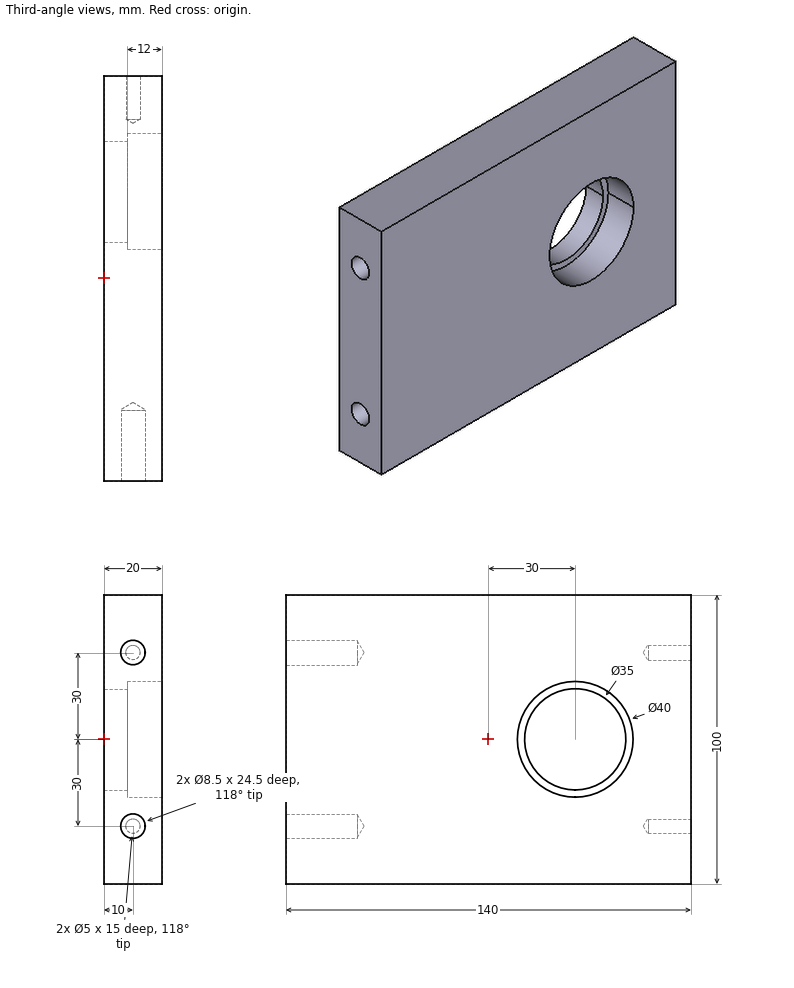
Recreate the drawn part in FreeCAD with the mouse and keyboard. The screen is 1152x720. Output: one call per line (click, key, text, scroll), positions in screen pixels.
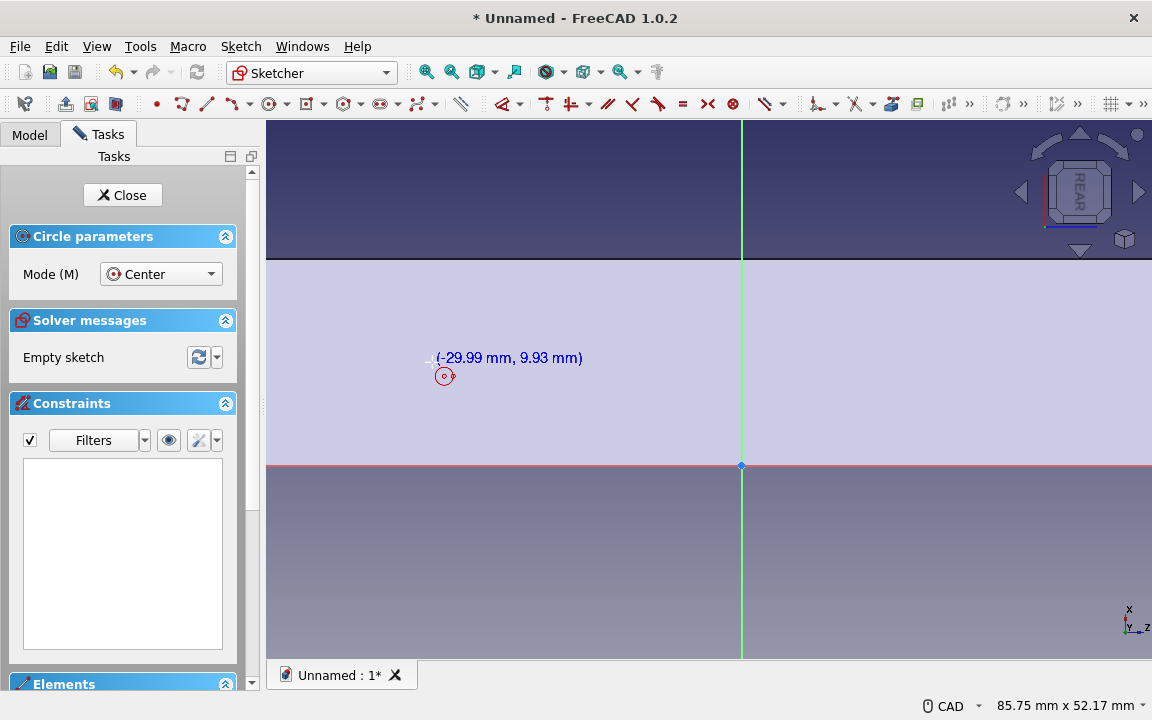
click(432, 363)
move(450, 344)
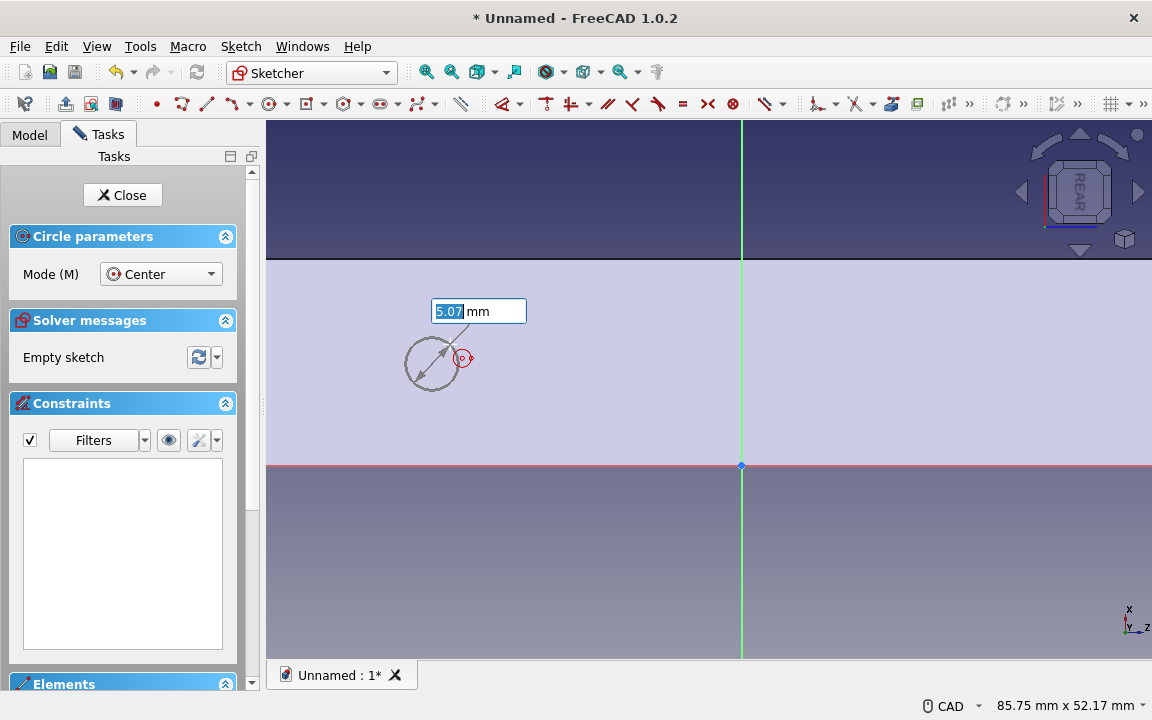
text(5)
key(Return)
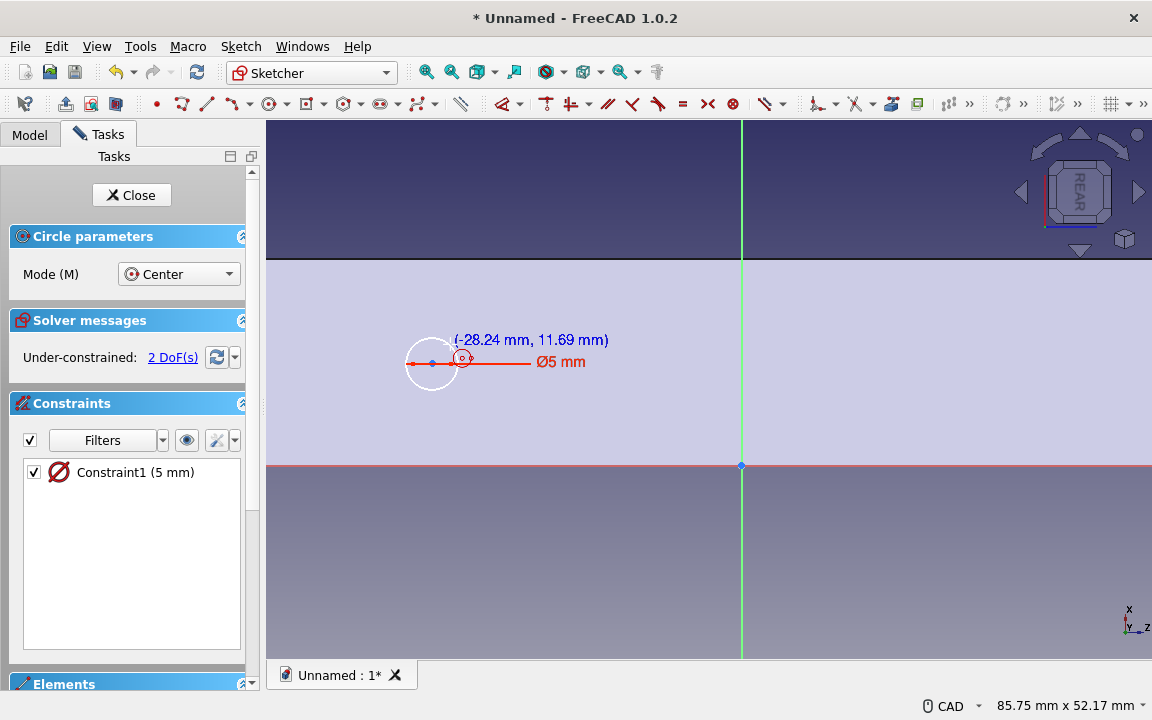
scroll(435, 366, down, 2)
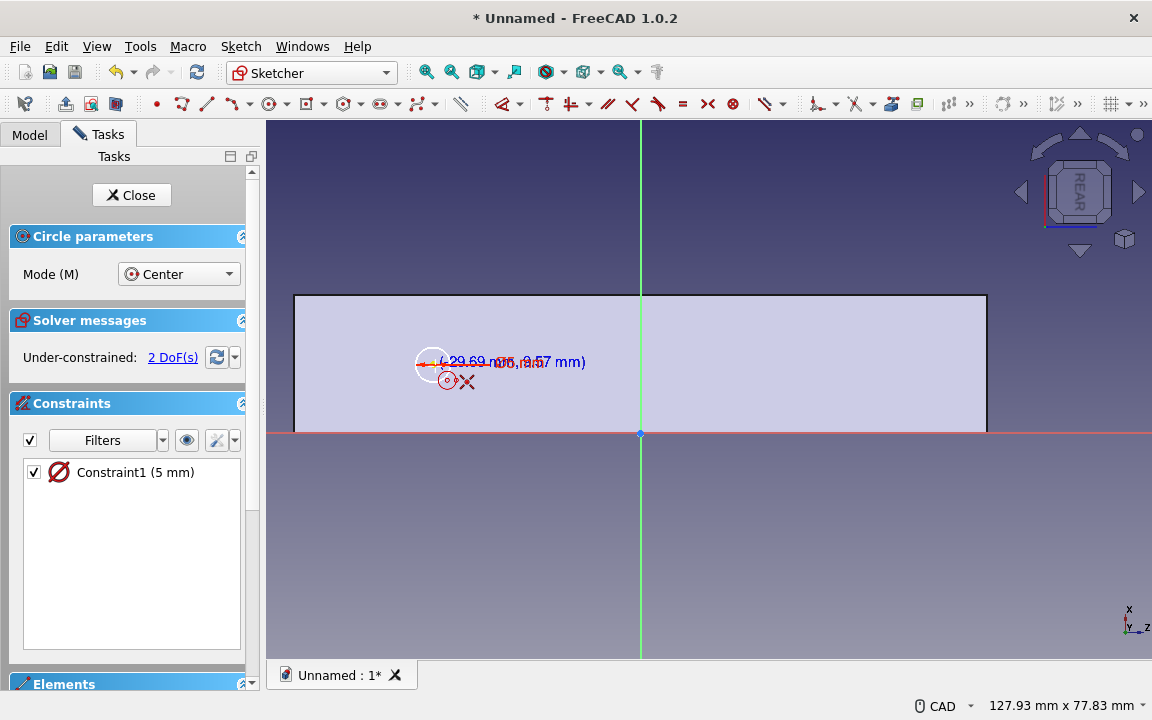
scroll(848, 364, up, 2)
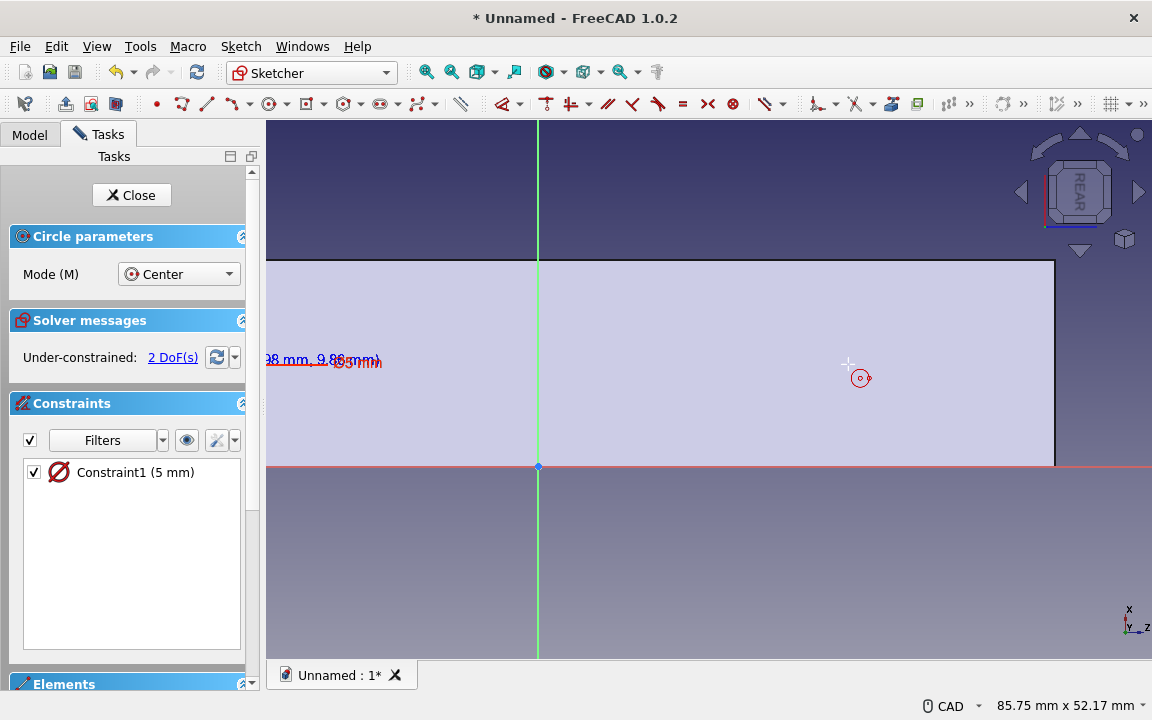
click(848, 363)
move(867, 345)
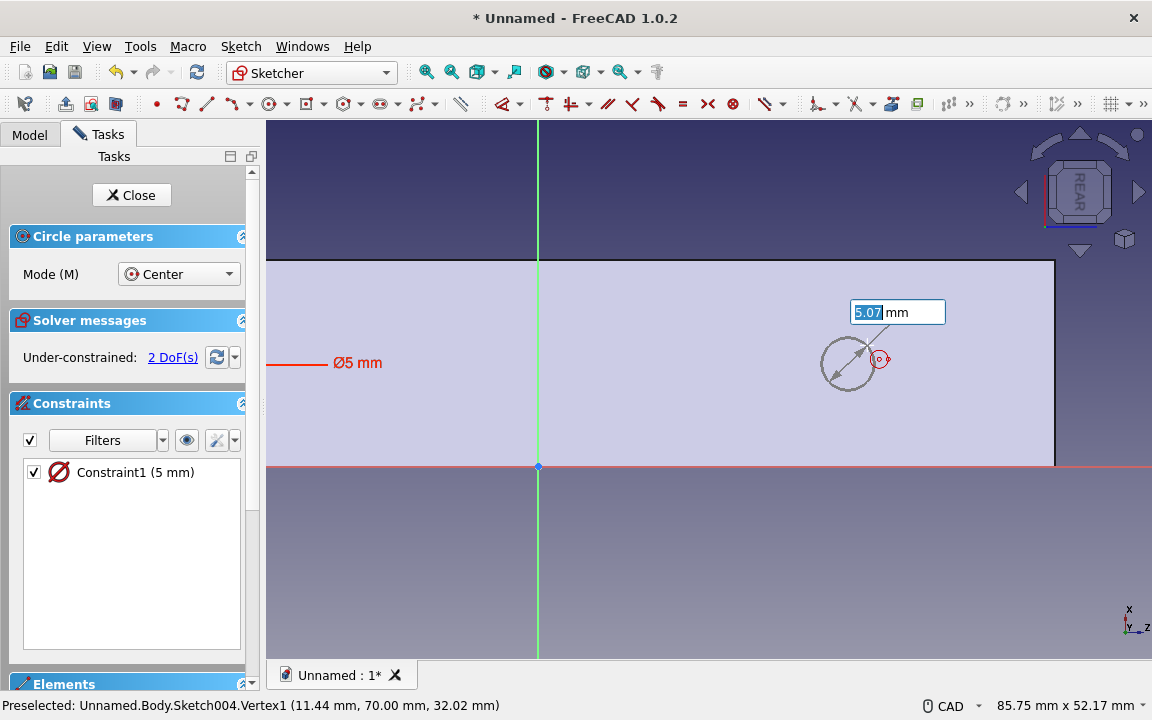
text(5)
key(Return)
key(Escape)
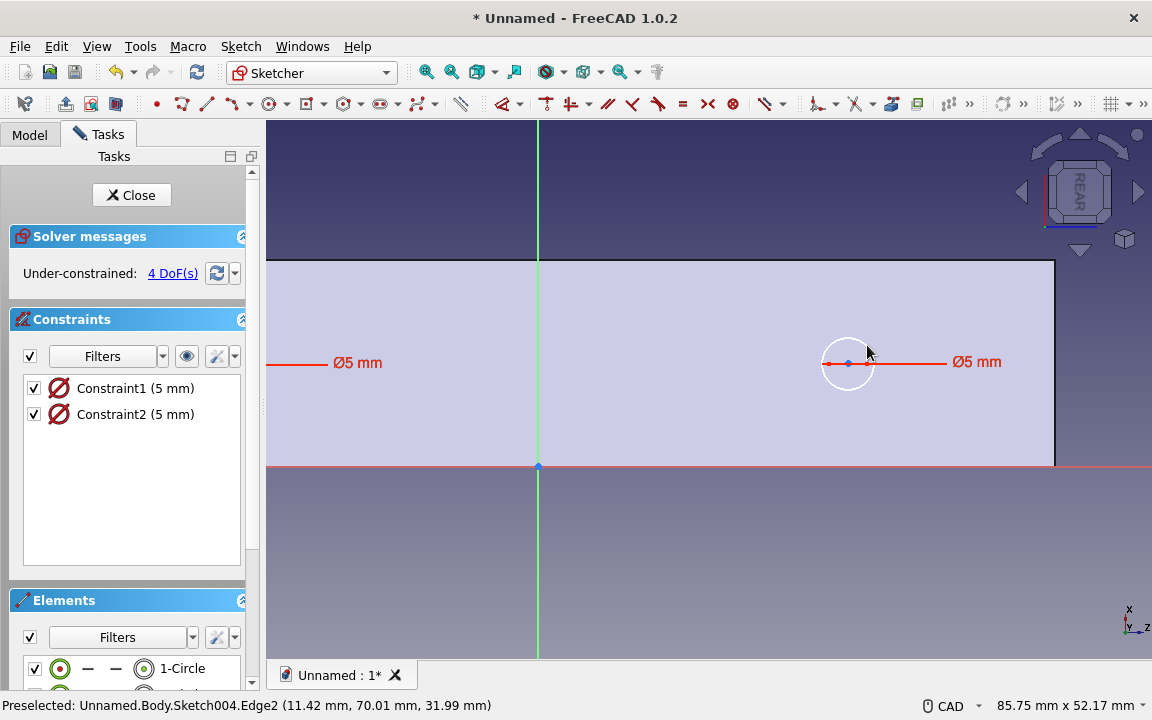
scroll(848, 364, down, 2)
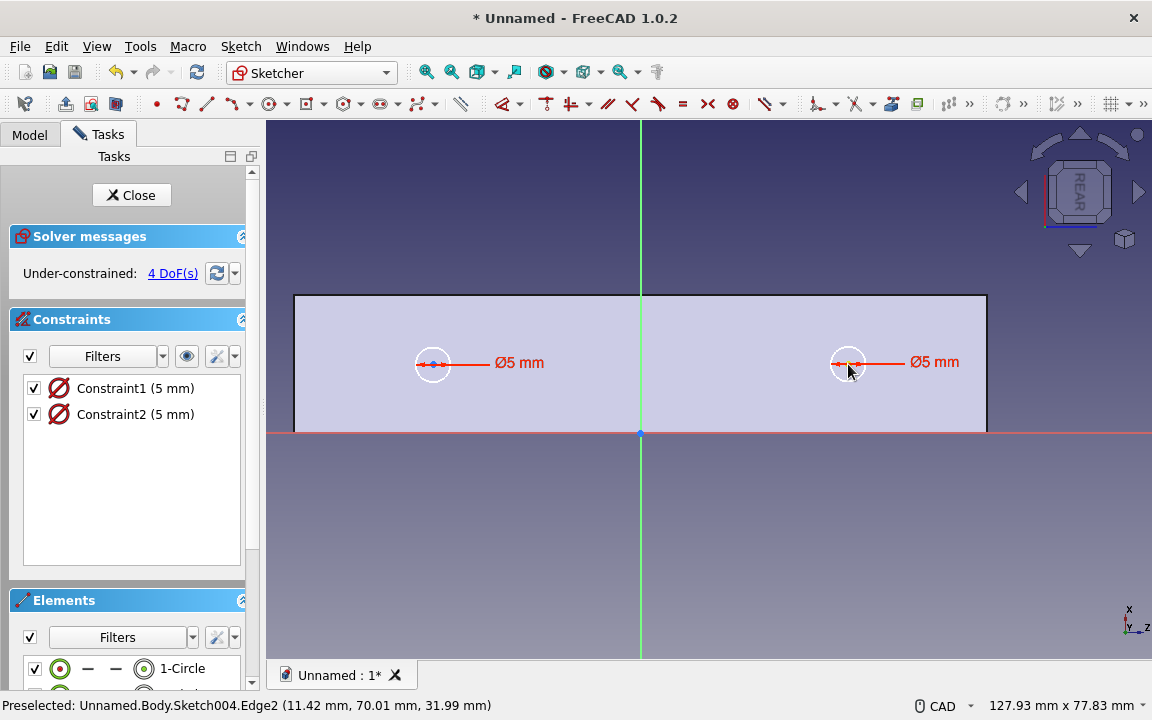
click(433, 365)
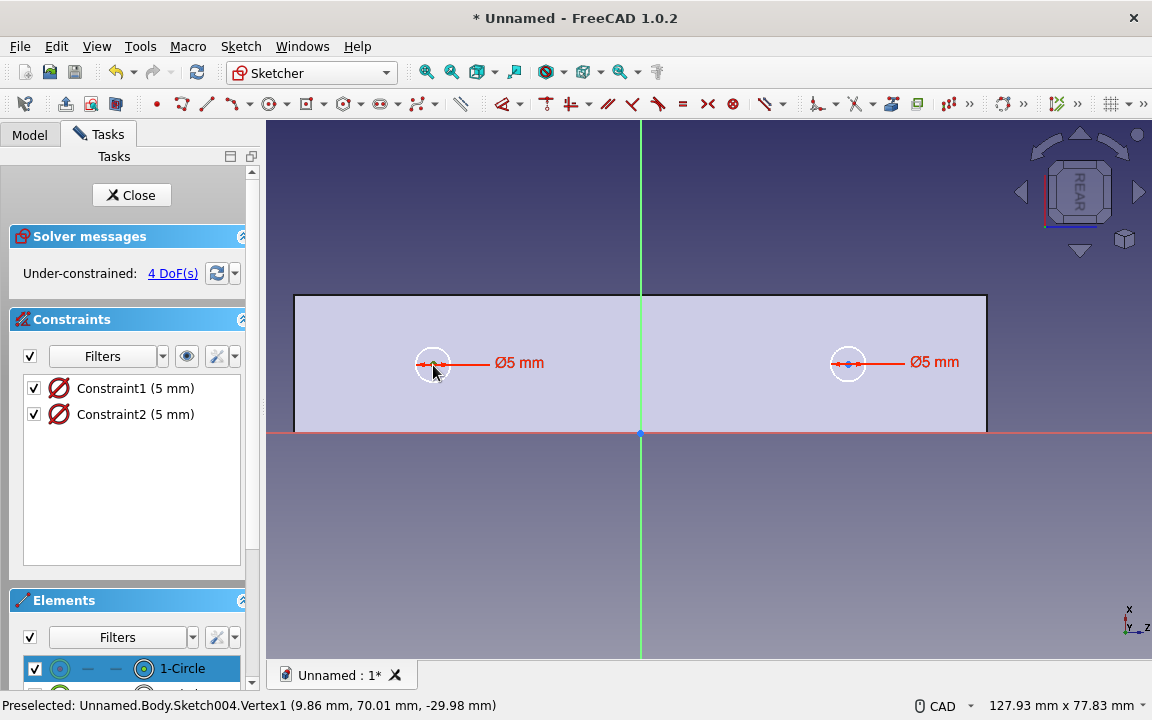
click(848, 364)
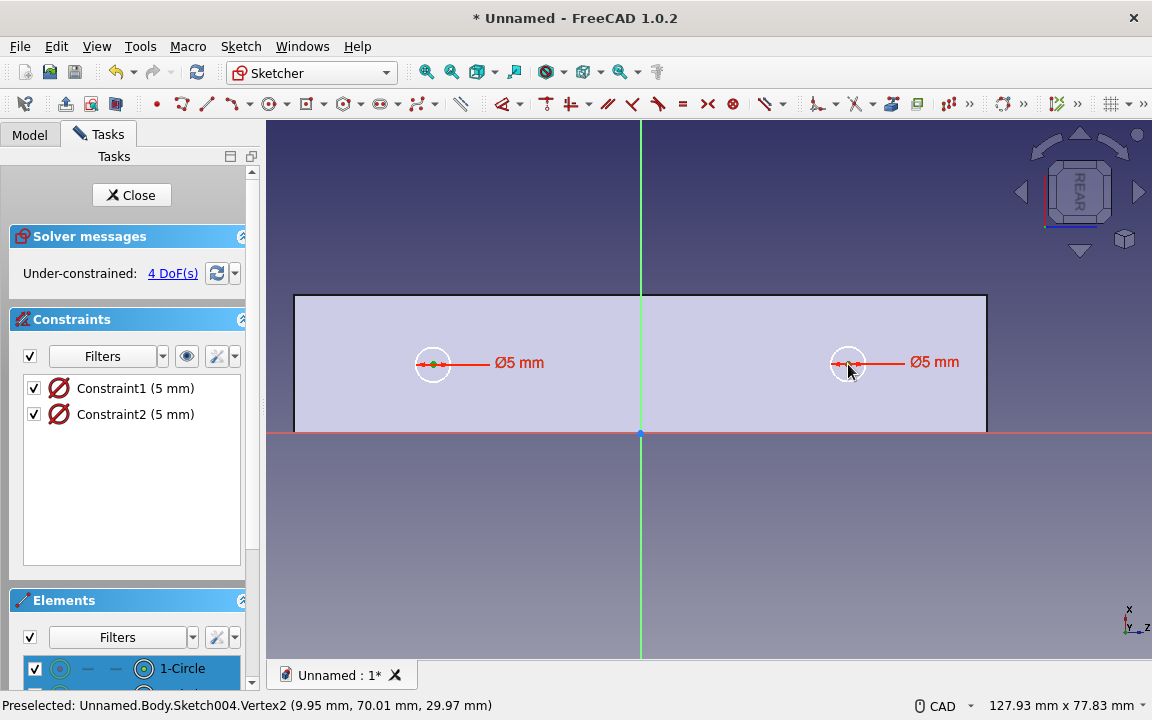
key(h)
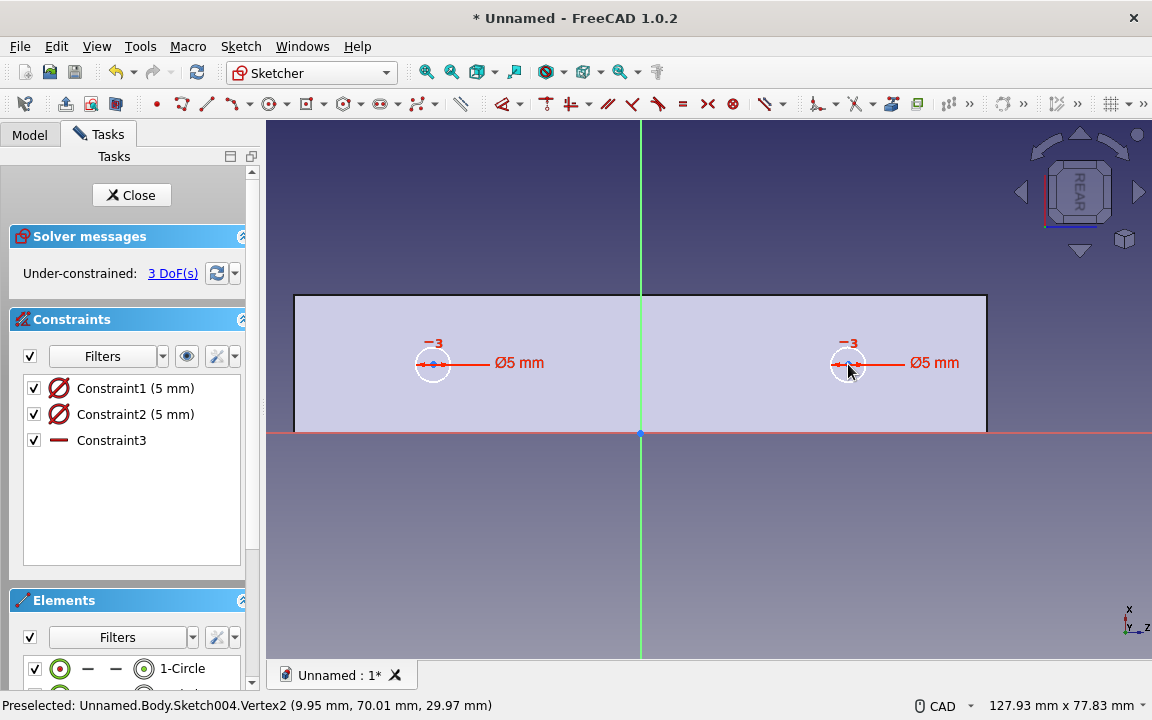
key(d)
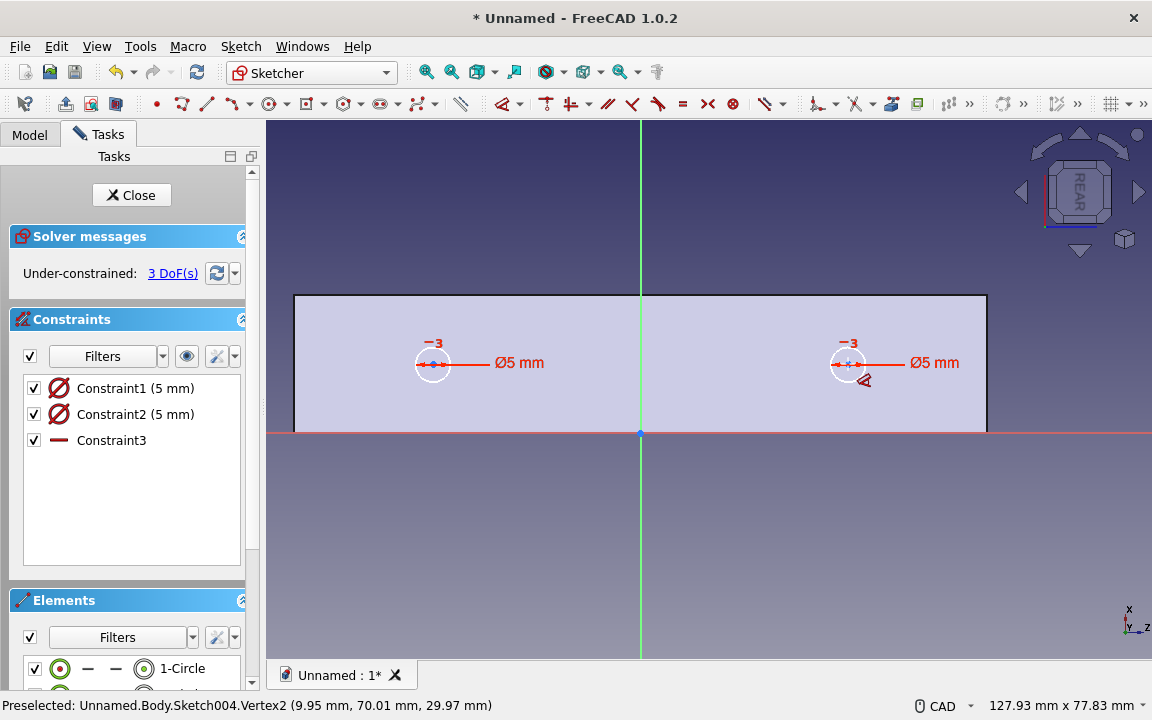
click(433, 365)
click(537, 467)